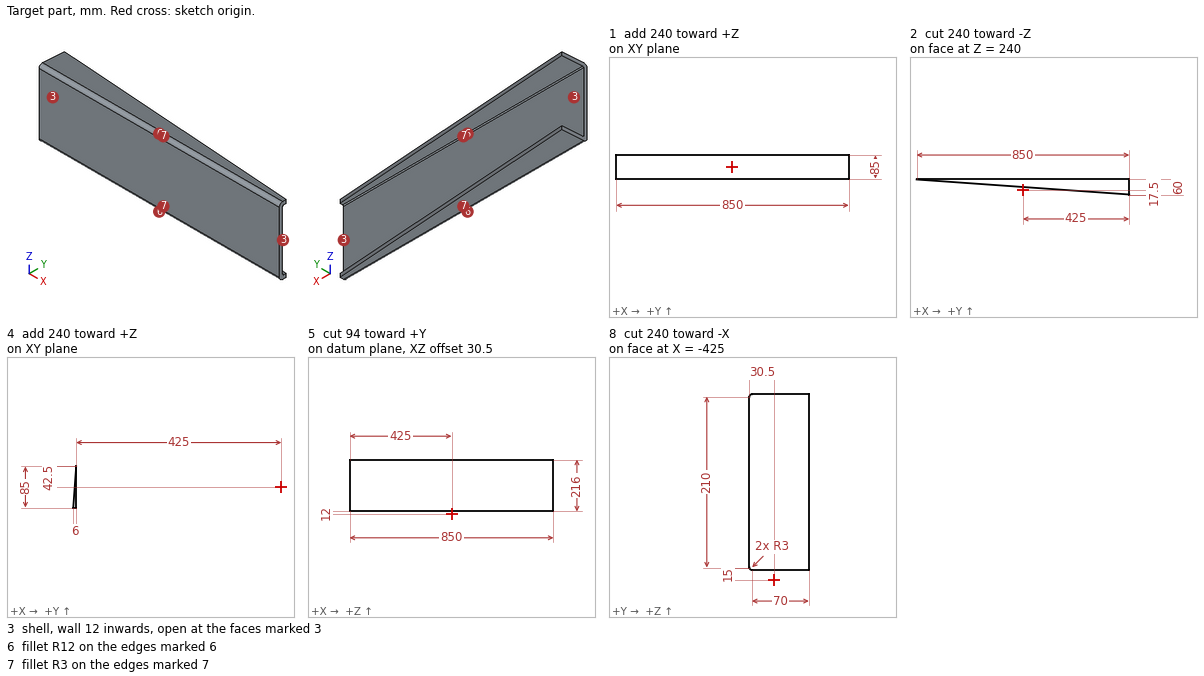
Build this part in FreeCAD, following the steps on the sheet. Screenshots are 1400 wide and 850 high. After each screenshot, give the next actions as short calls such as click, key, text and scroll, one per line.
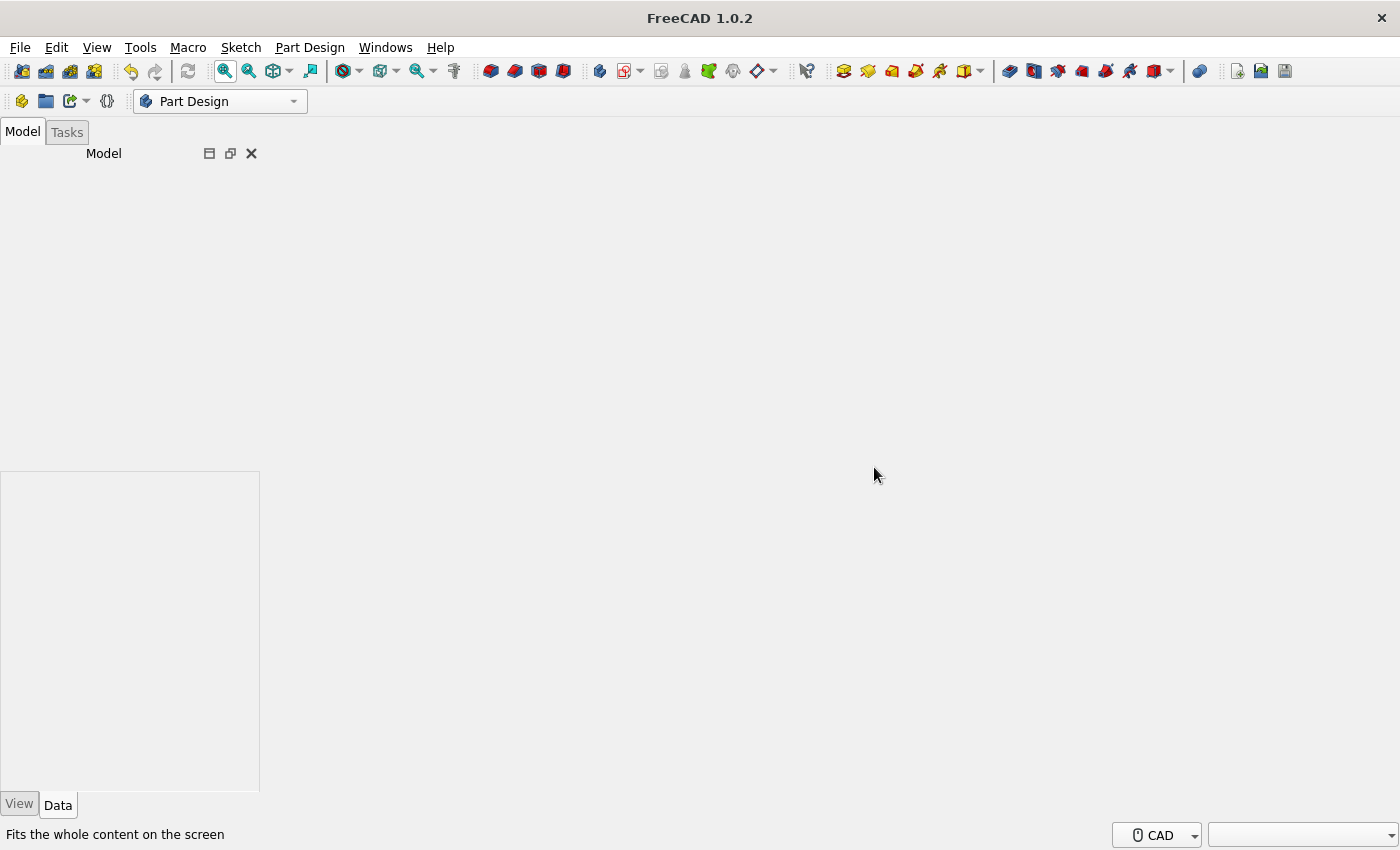
key(ctrl+n)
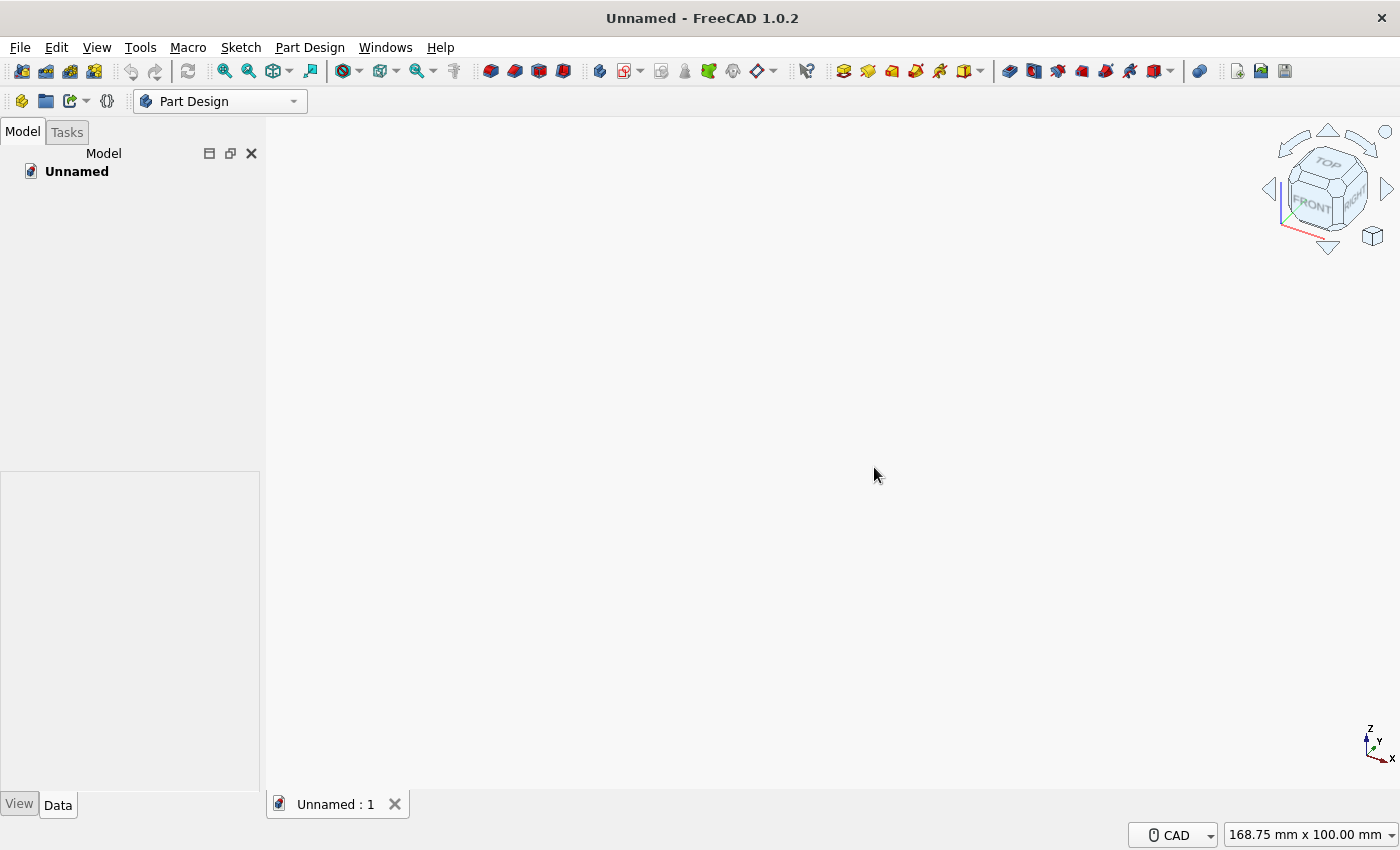
click(624, 72)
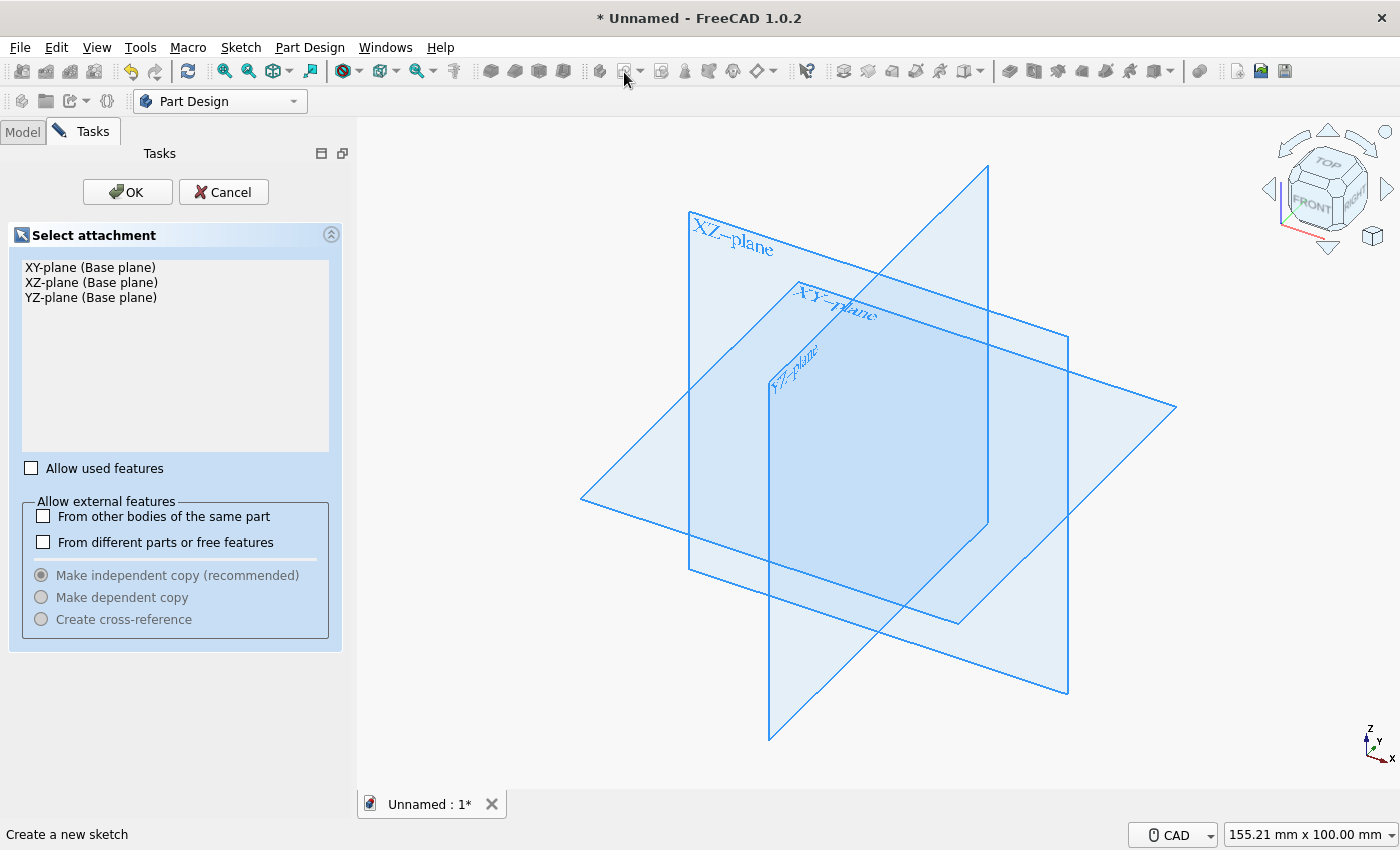
click(82, 268)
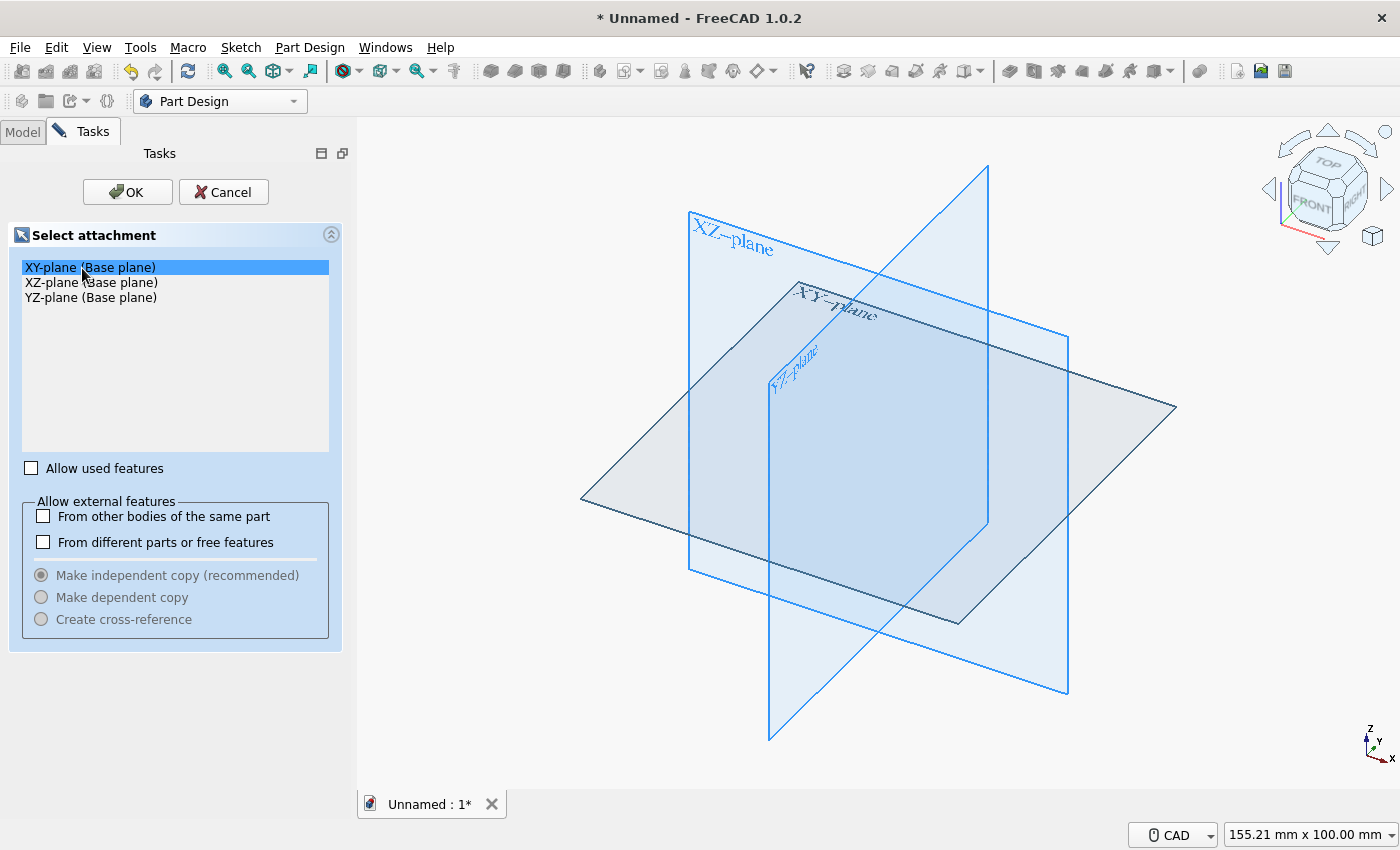
click(128, 192)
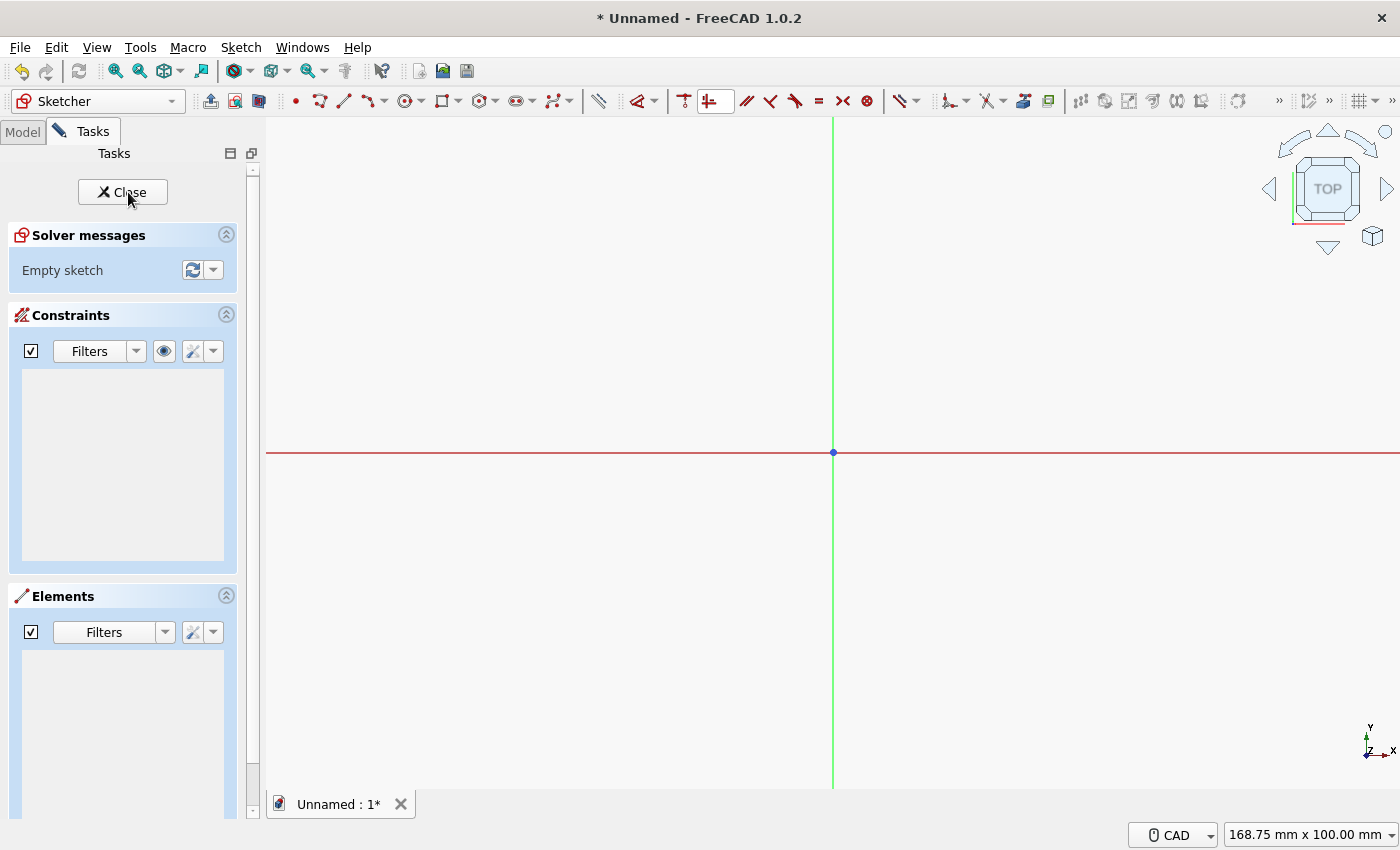
scroll(756, 453, down, 11)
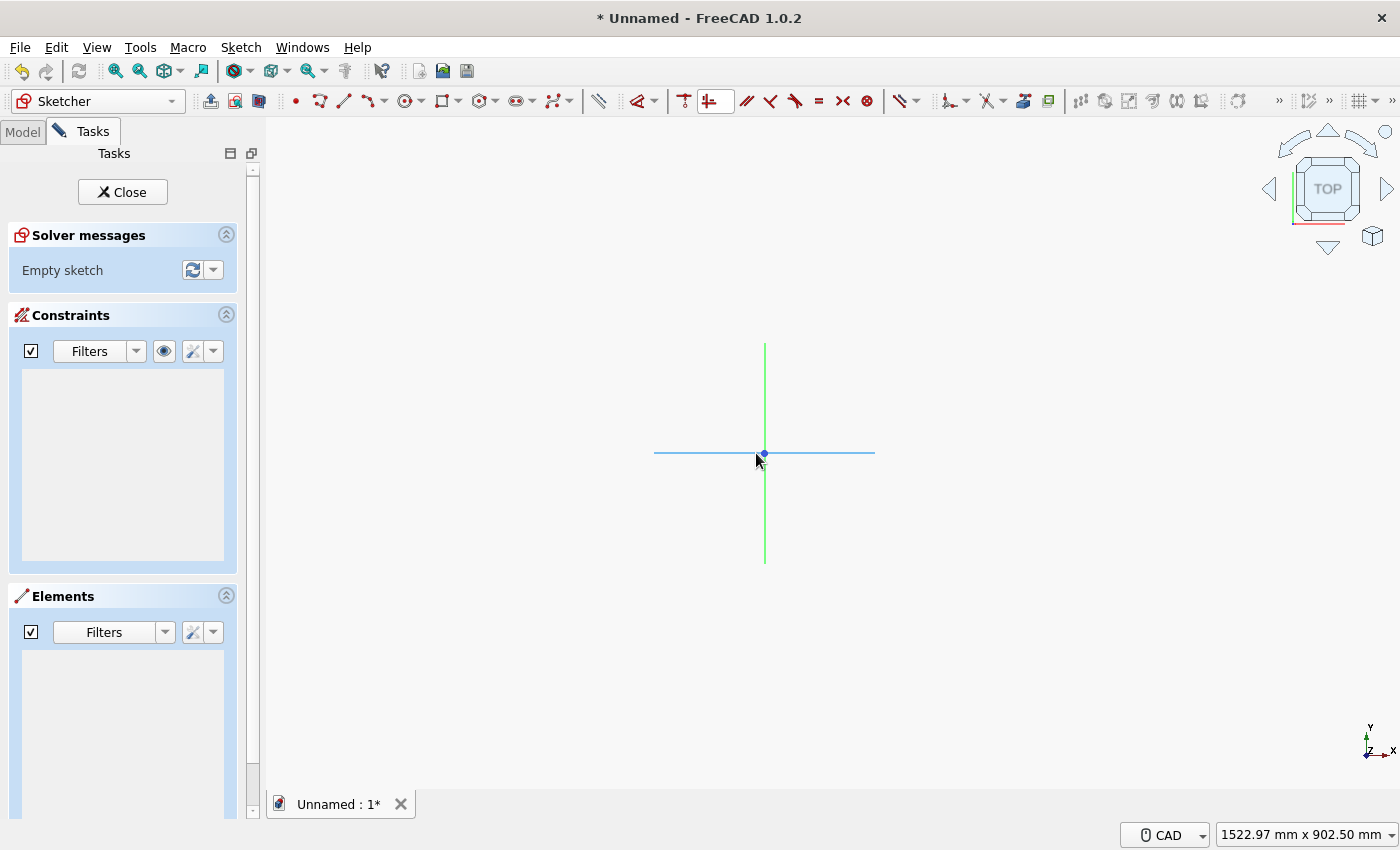
key(g)
key(v)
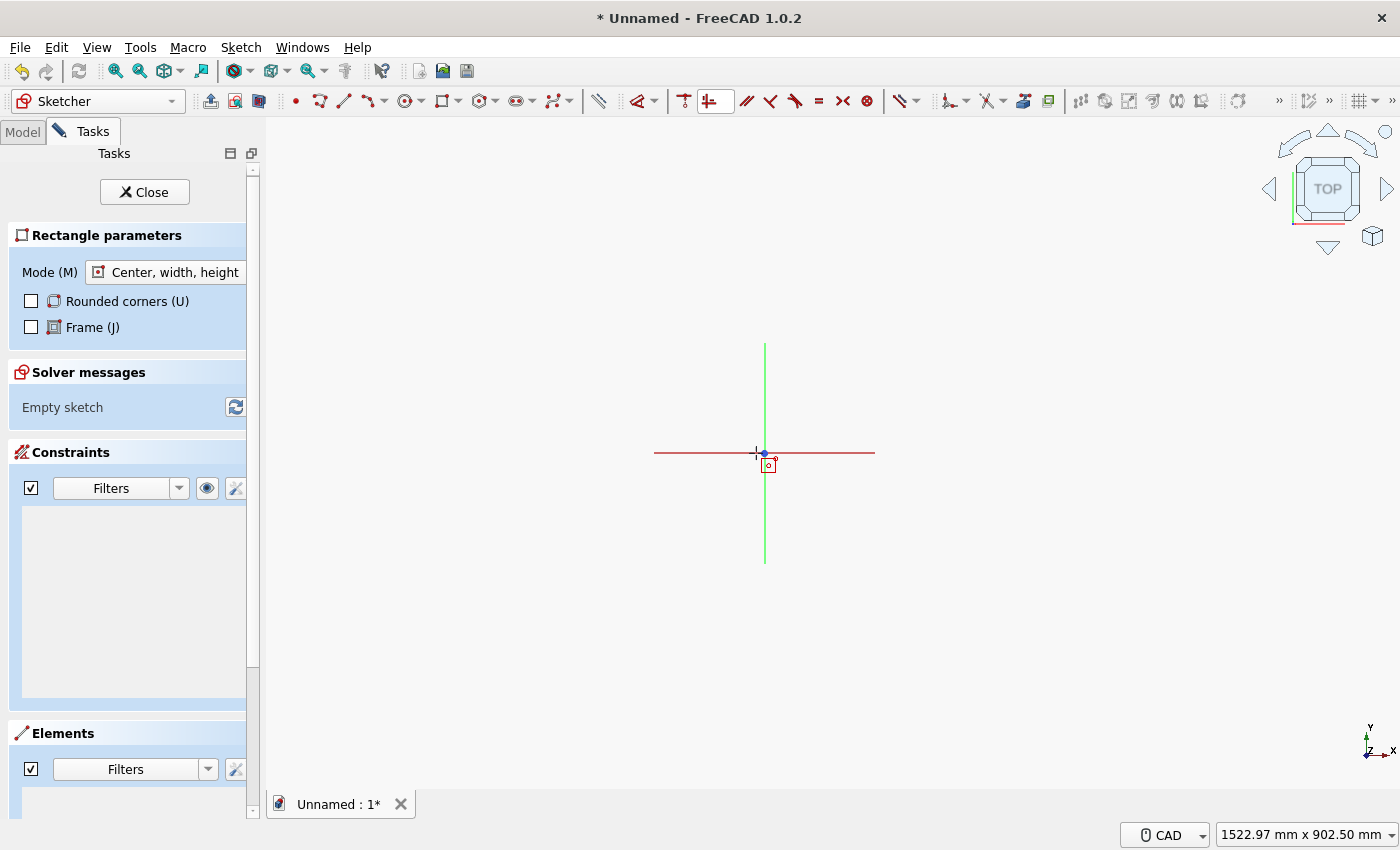
click(765, 453)
move(1081, 422)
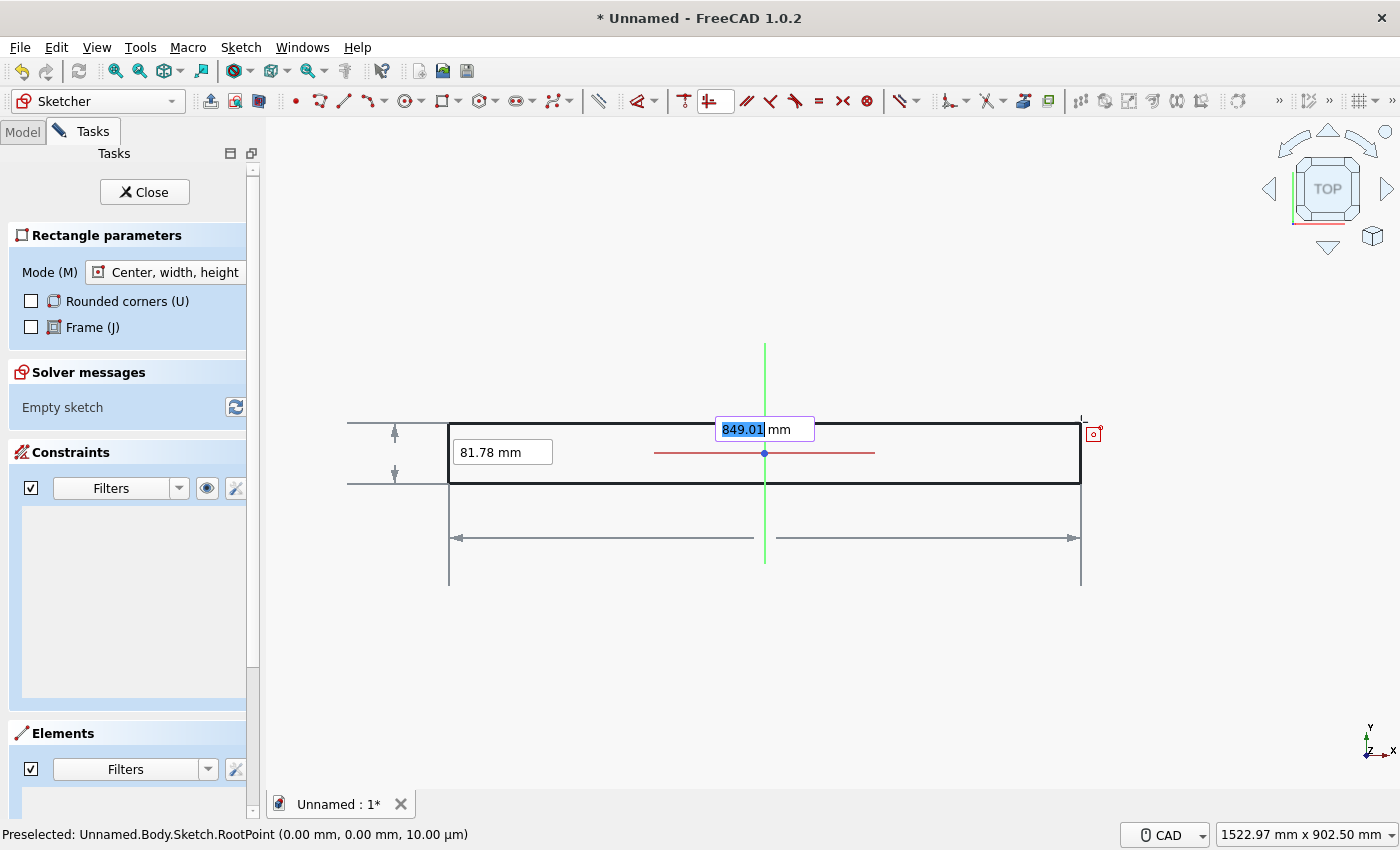
text(850)
key(Tab)
text(85)
key(Return)
key(Escape)